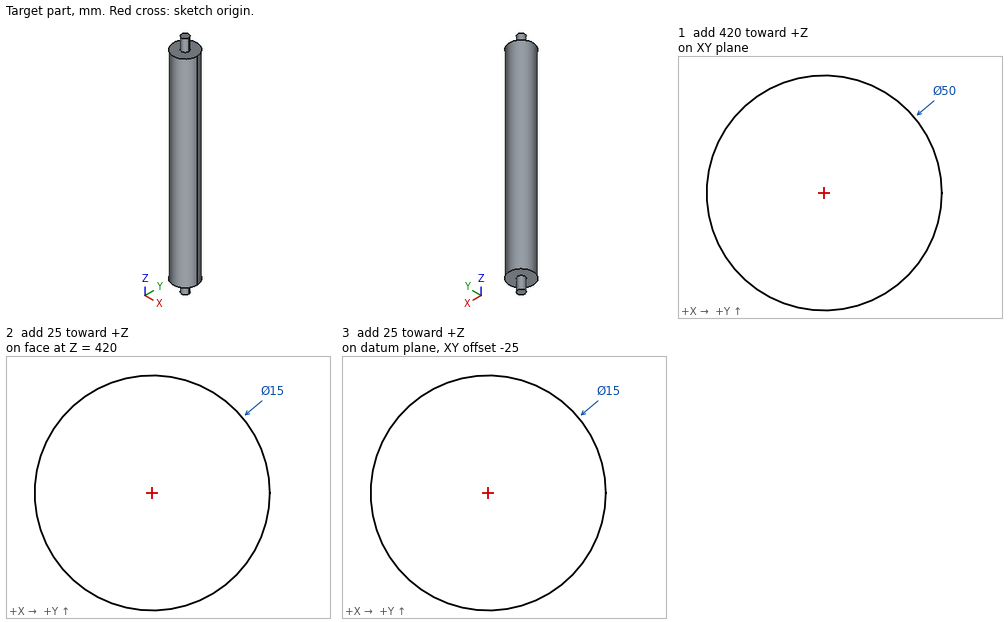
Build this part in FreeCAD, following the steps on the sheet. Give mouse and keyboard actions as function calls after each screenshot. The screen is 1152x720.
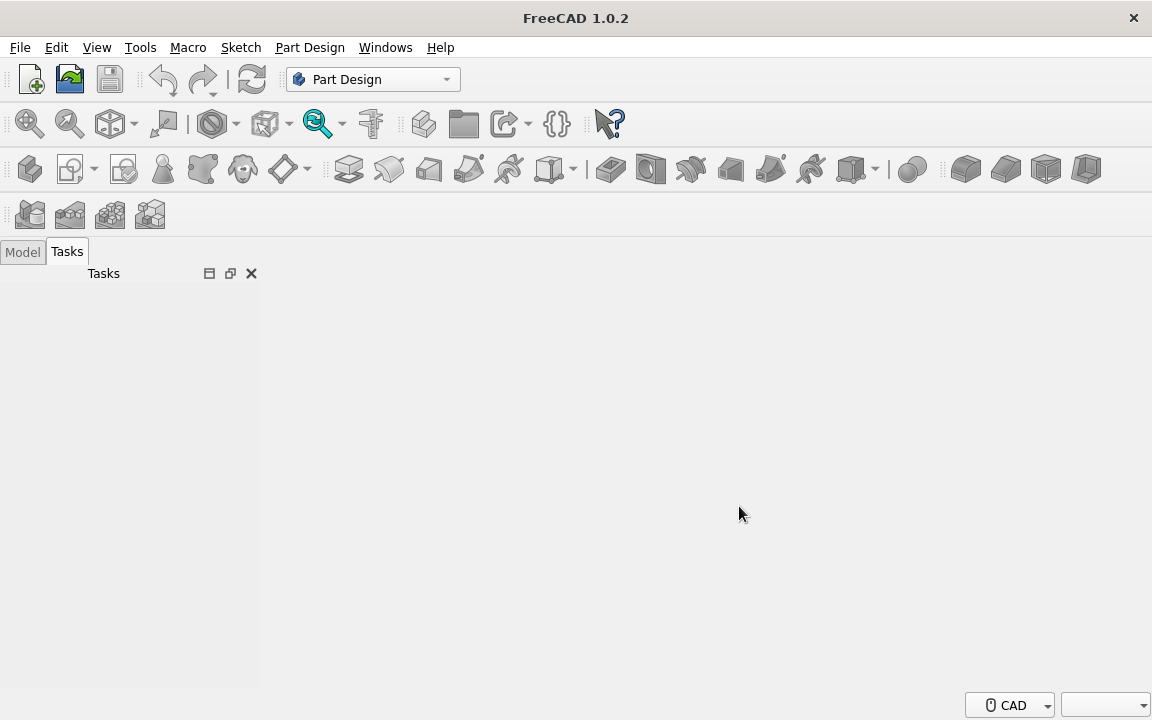
key(ctrl+n)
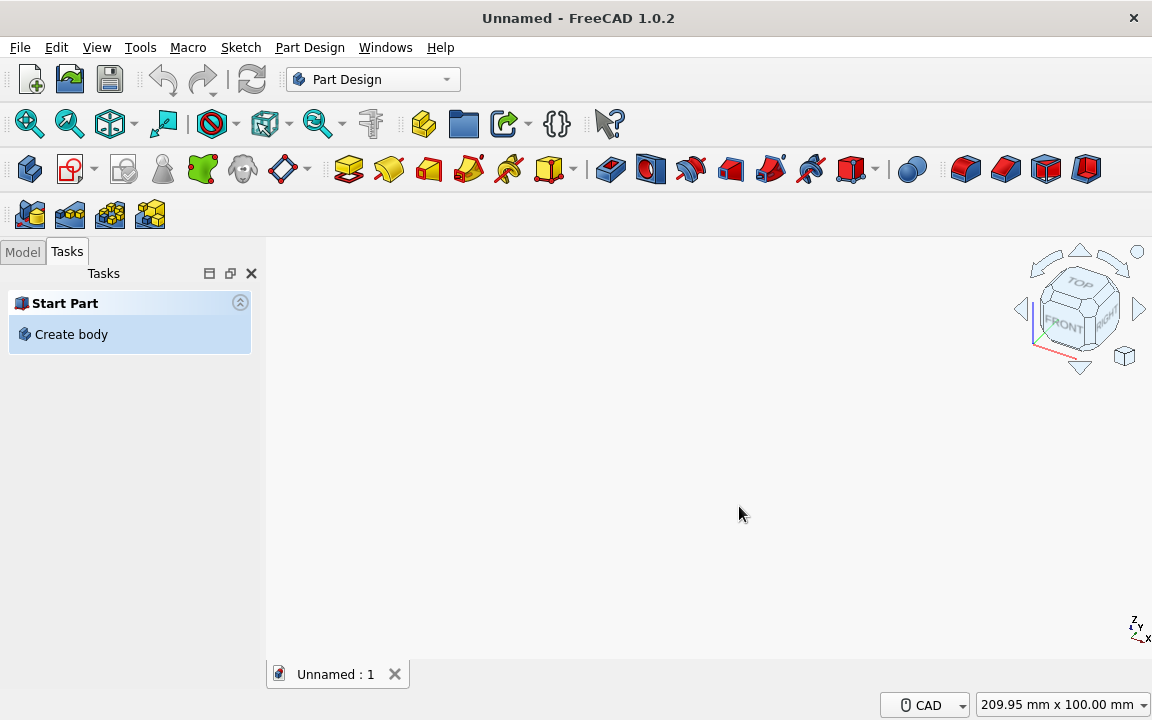
click(70, 170)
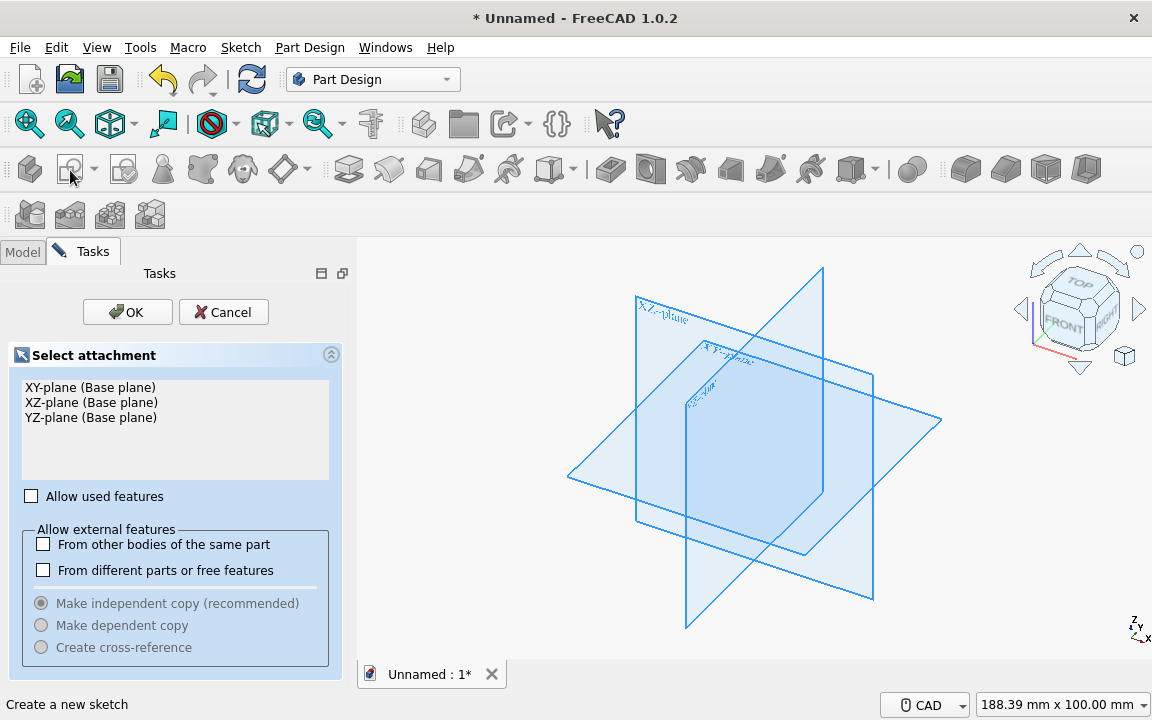
click(82, 388)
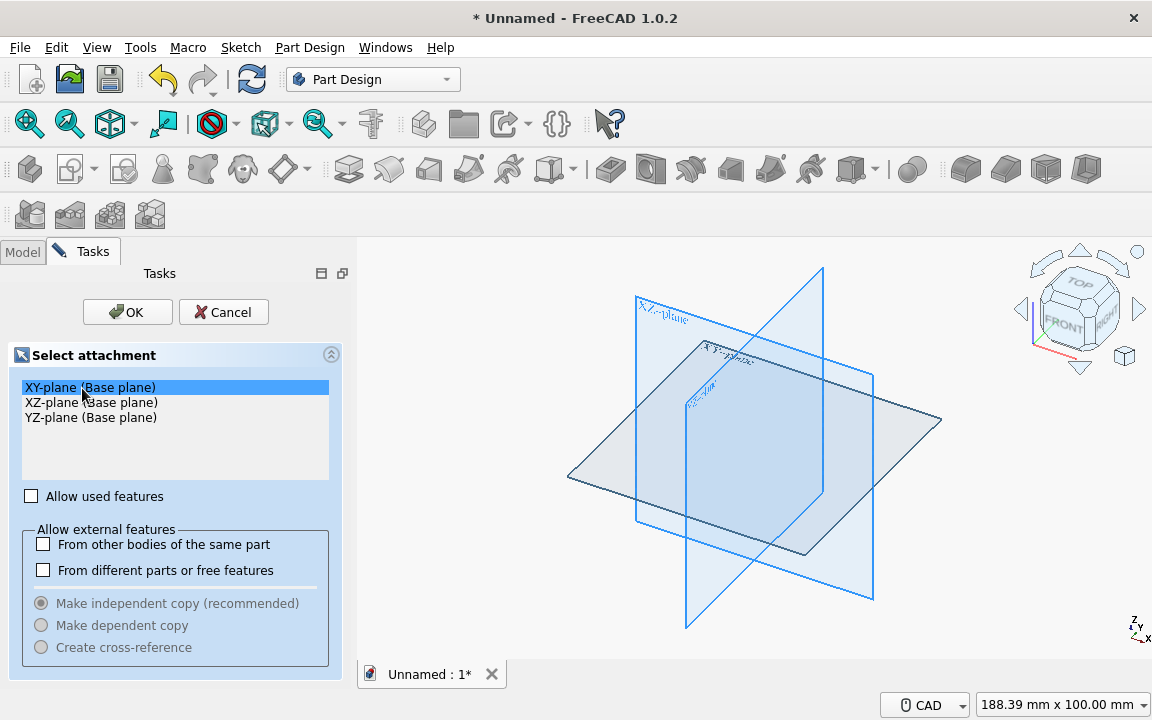
click(128, 312)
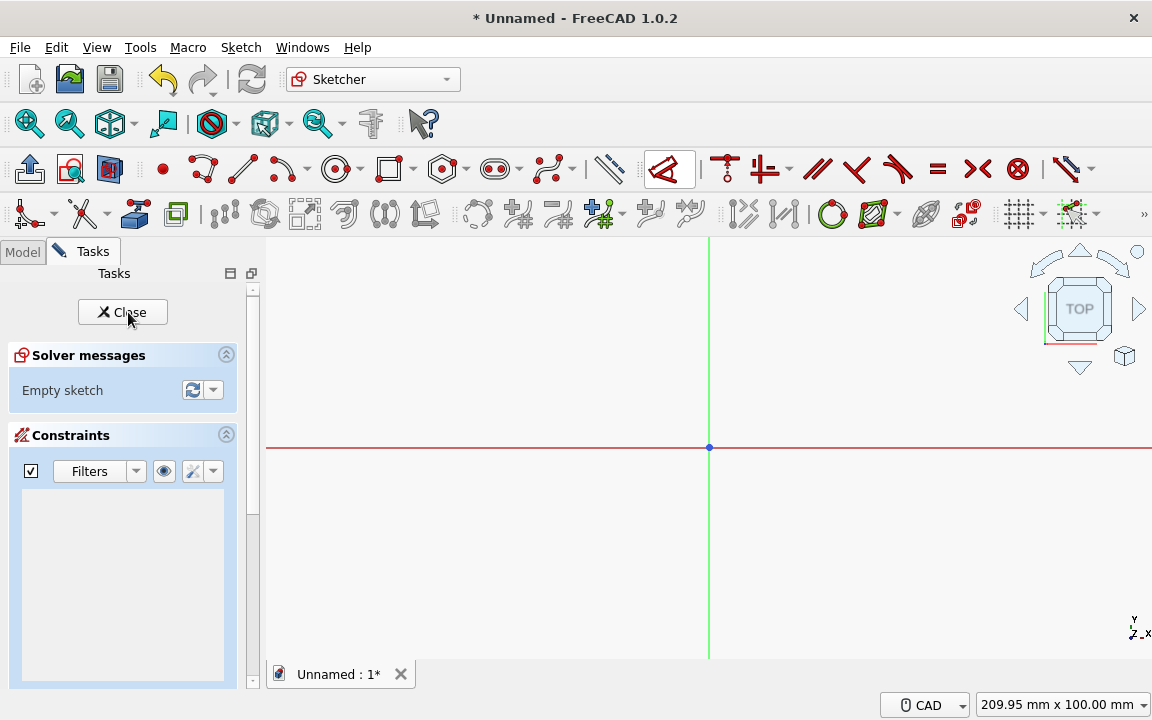
click(336, 170)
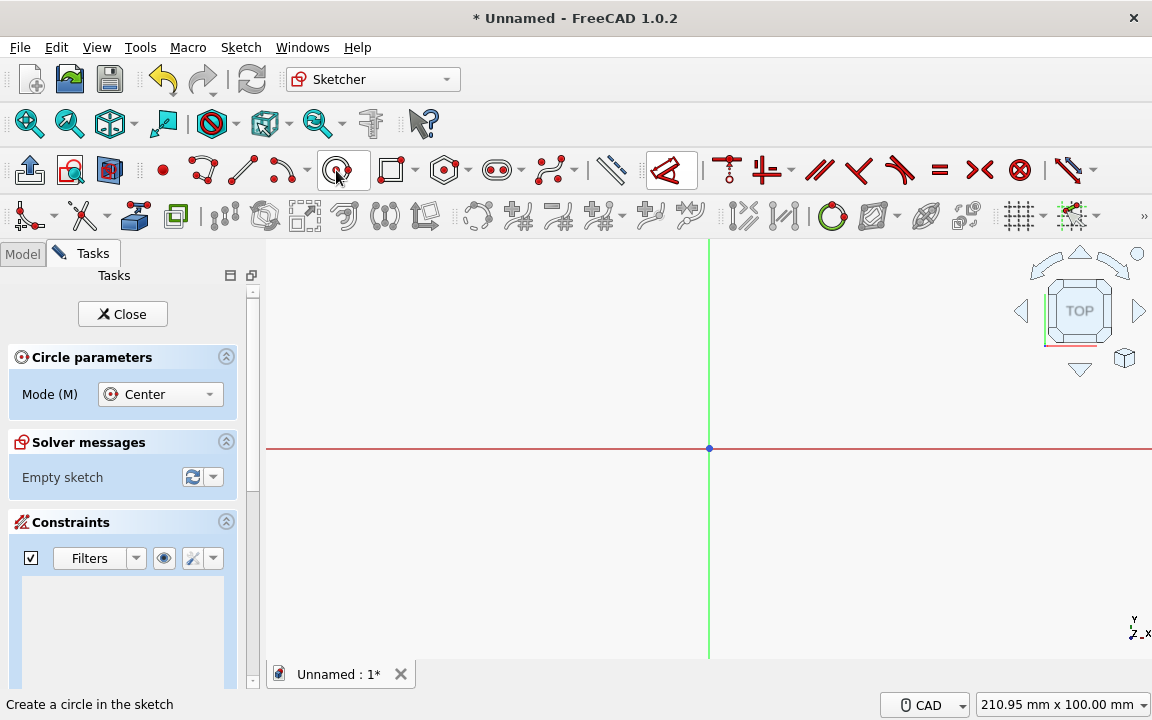
click(709, 449)
click(783, 375)
key(Escape)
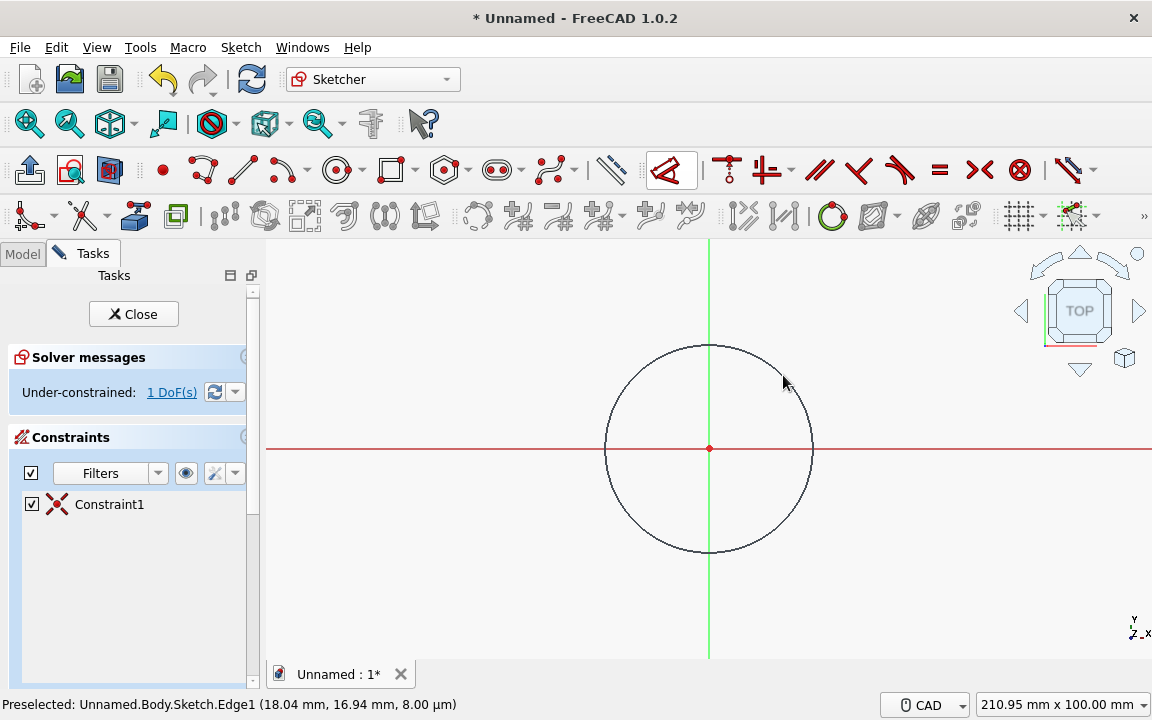
key(d)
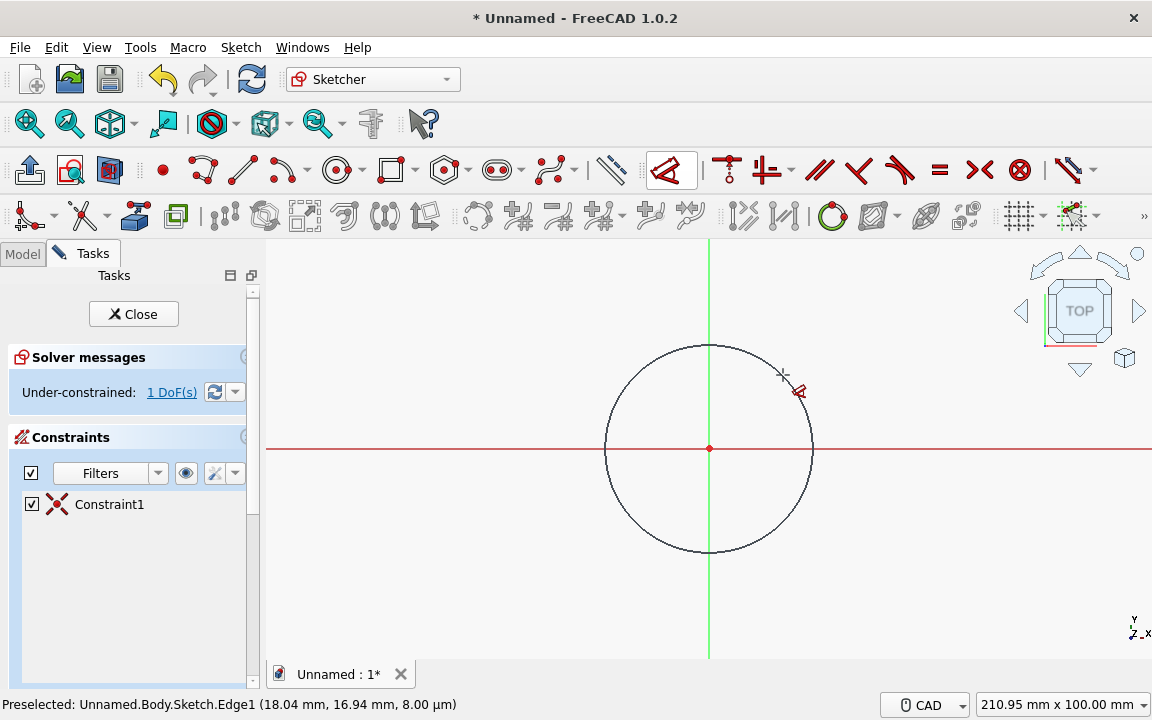
click(782, 375)
click(804, 352)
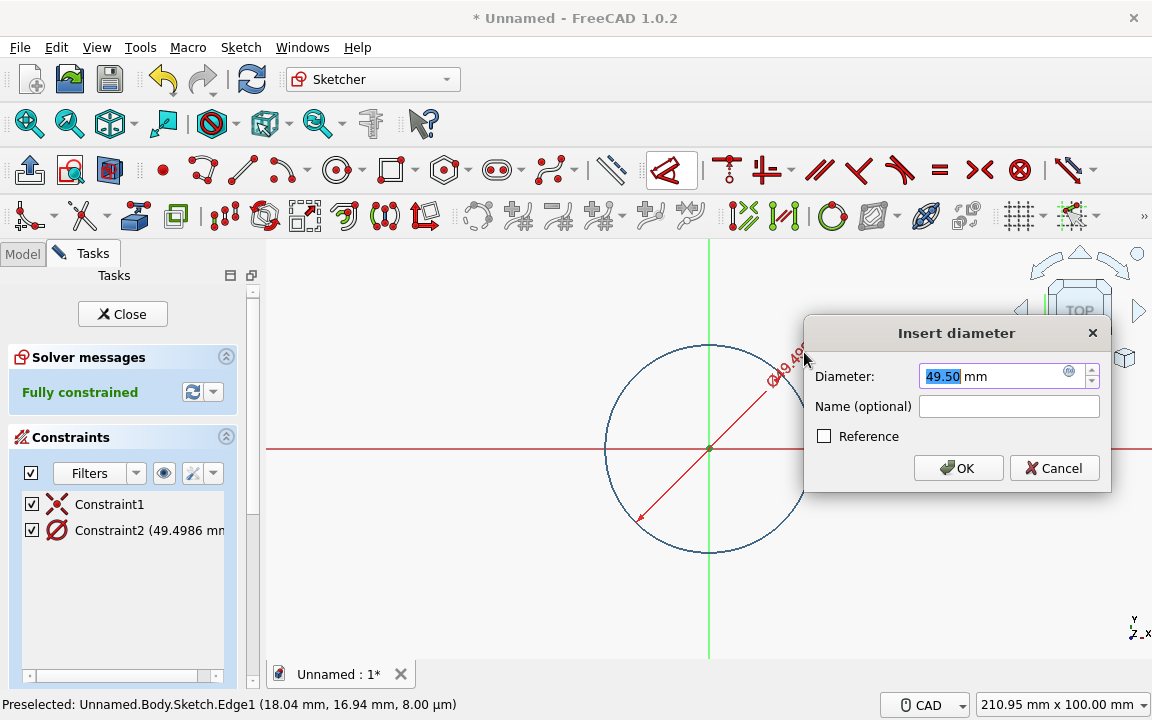
text(50)
key(Return)
key(Escape)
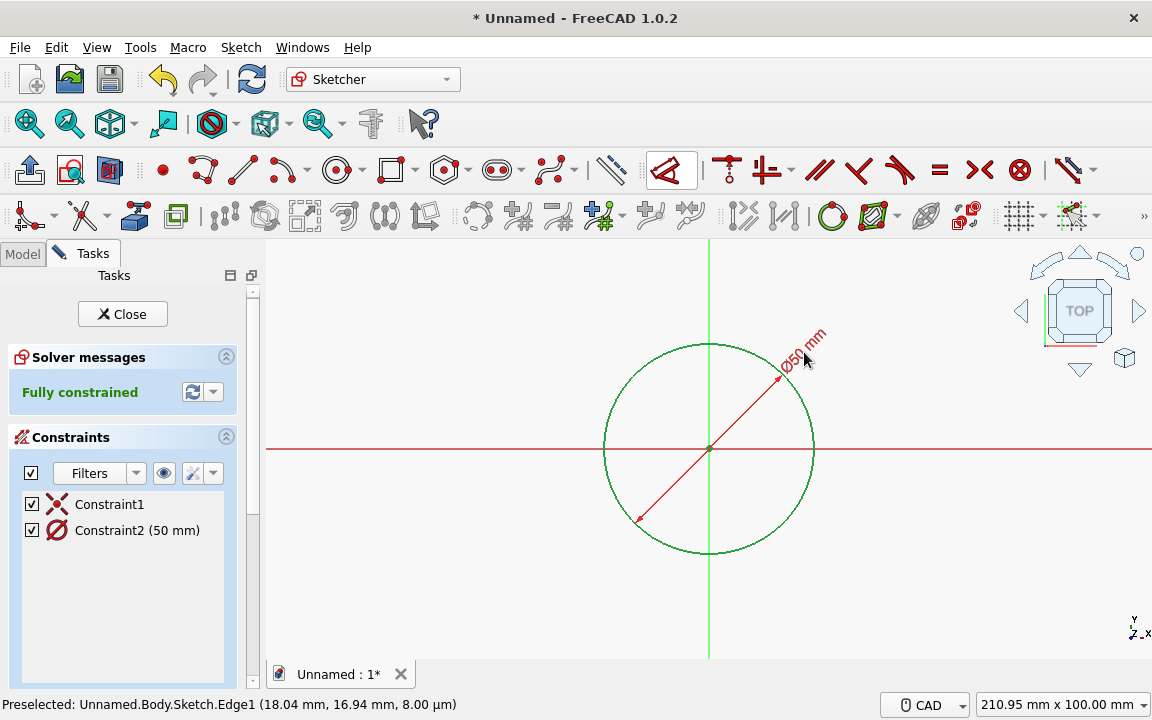
click(123, 314)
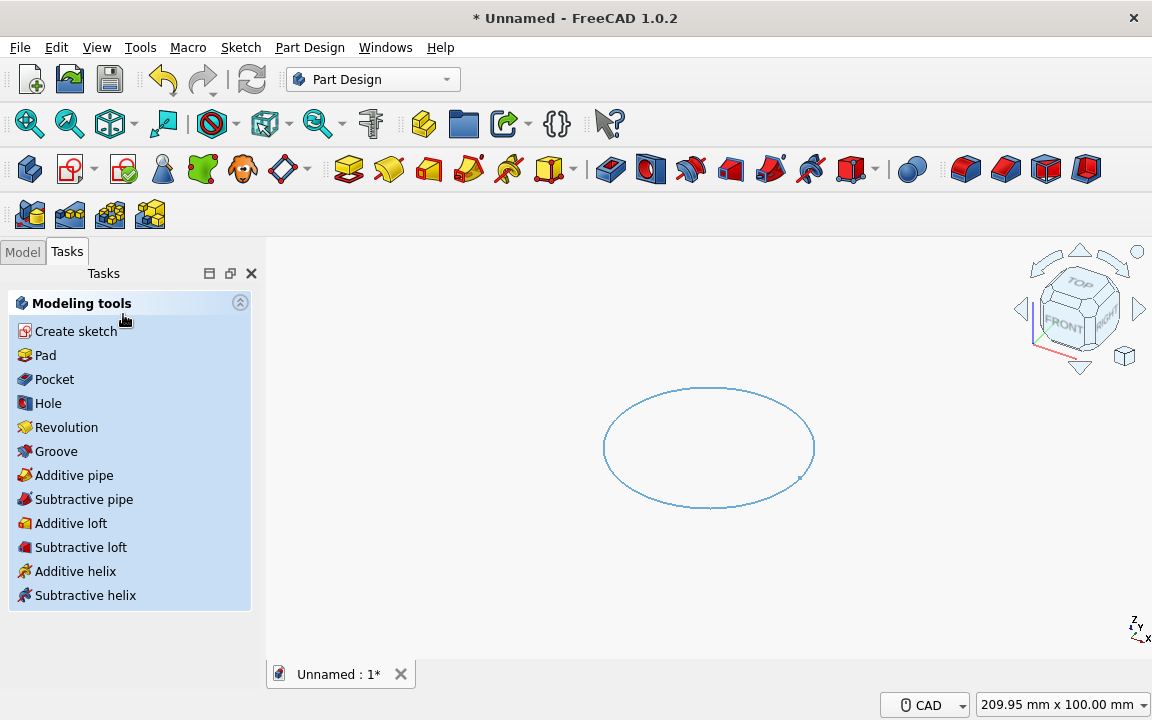
click(350, 170)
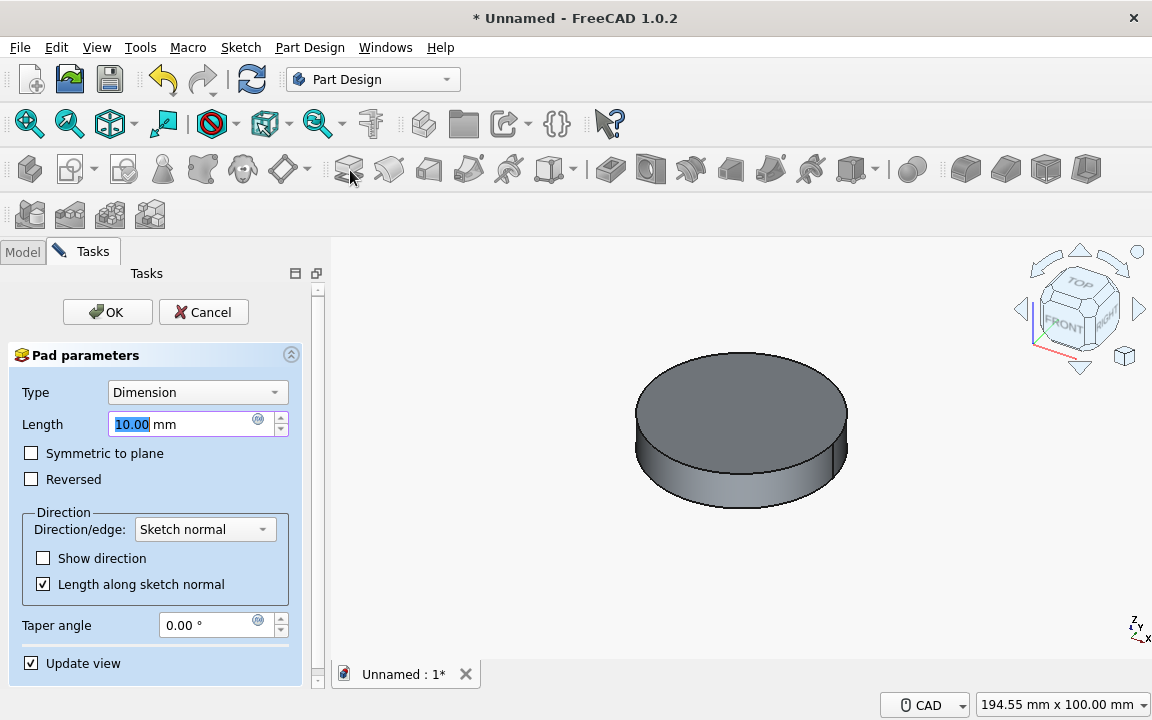
text(420)
key(Tab)